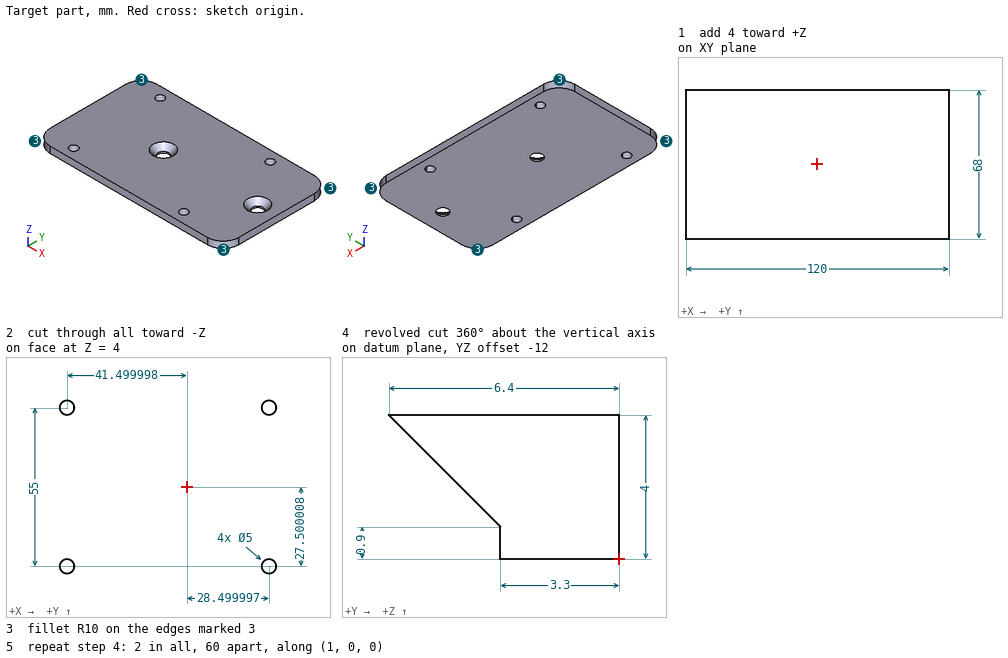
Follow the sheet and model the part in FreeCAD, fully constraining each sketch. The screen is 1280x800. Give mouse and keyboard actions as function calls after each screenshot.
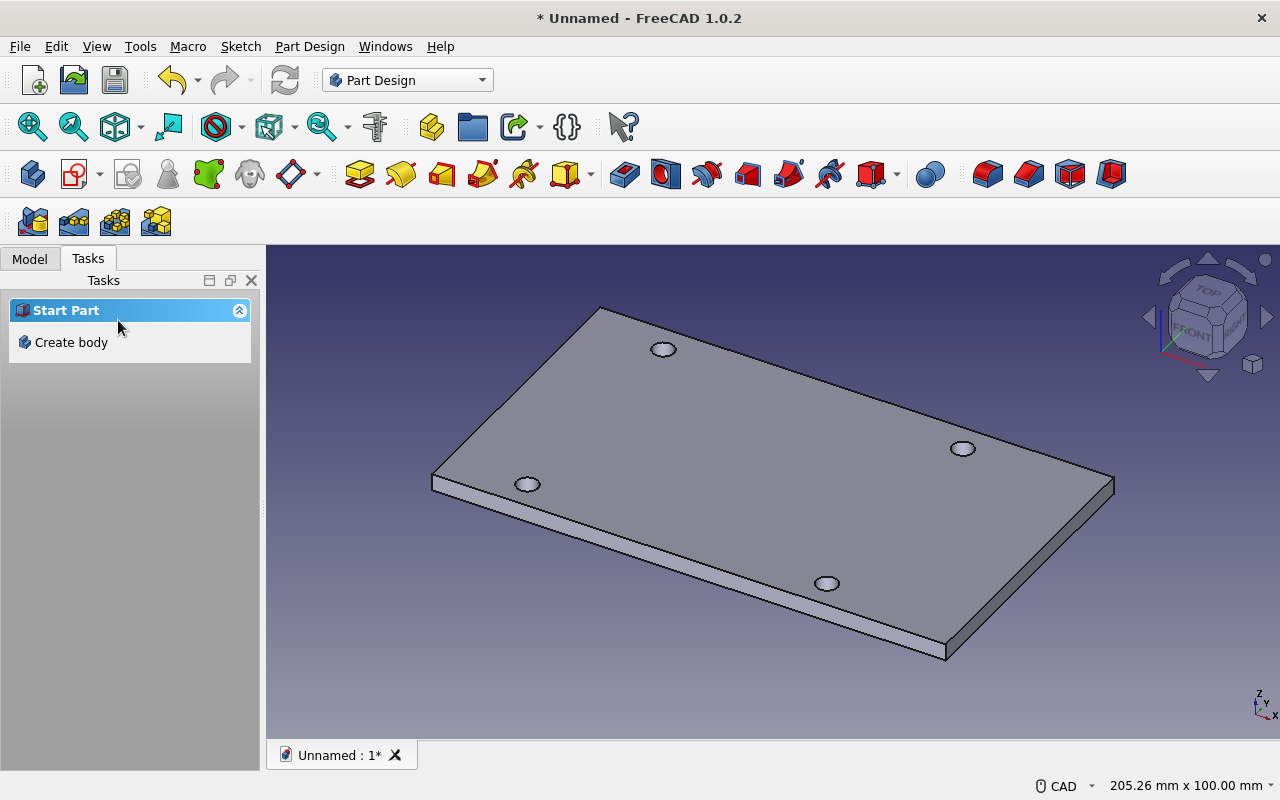
click(946, 651)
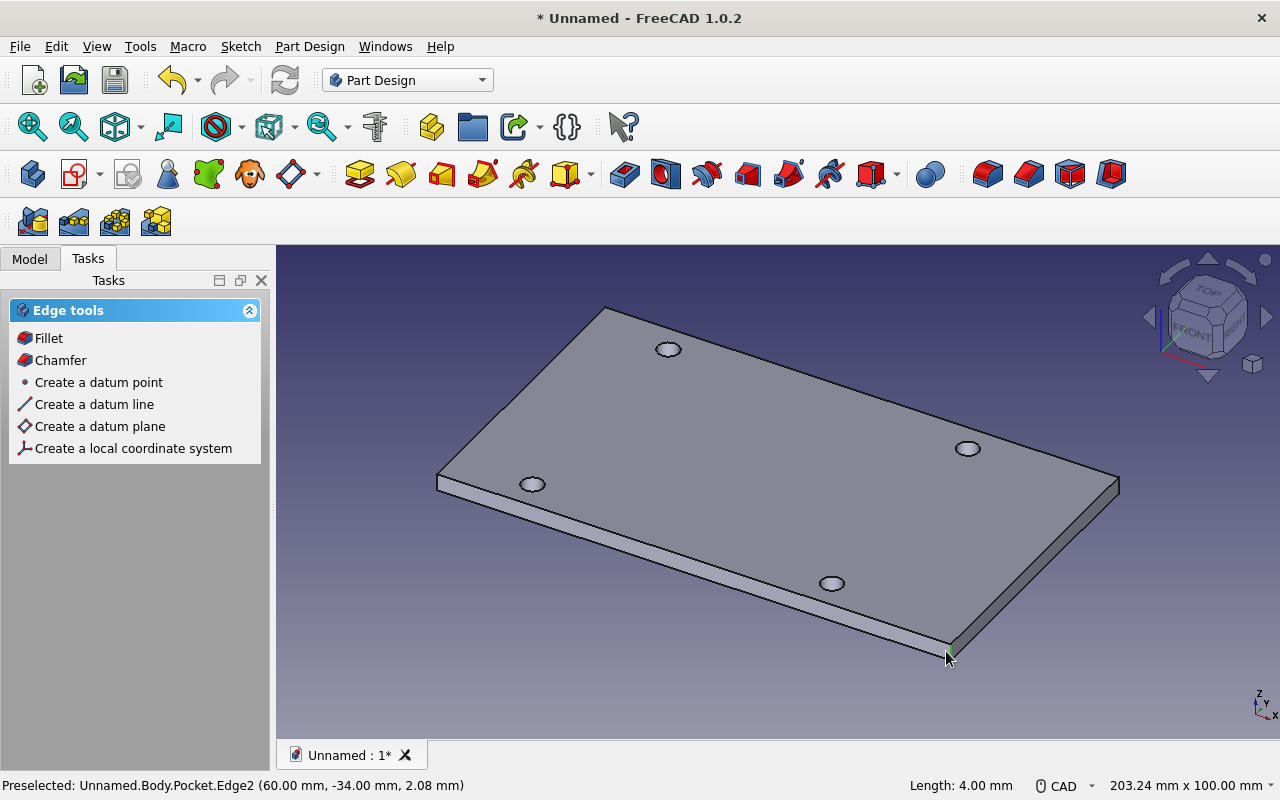
scroll(437, 481, up, 4)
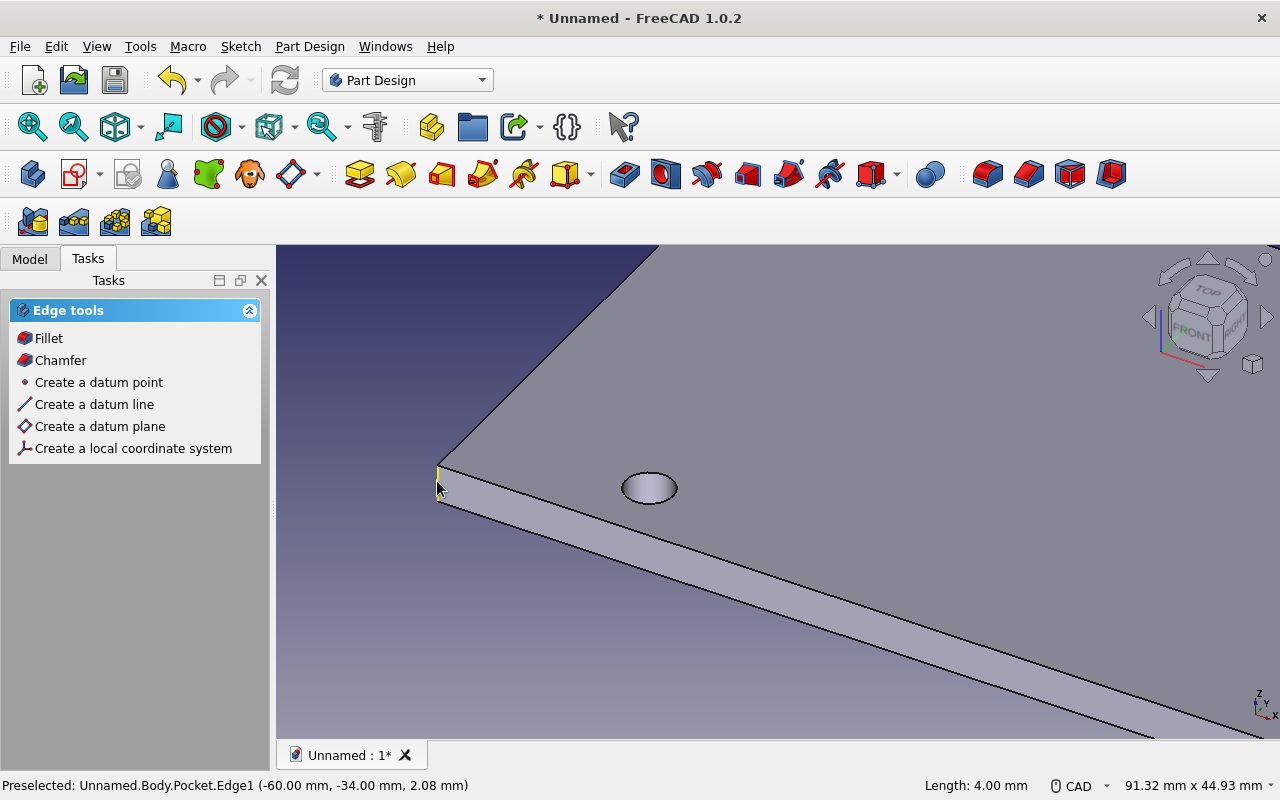
click(33, 128)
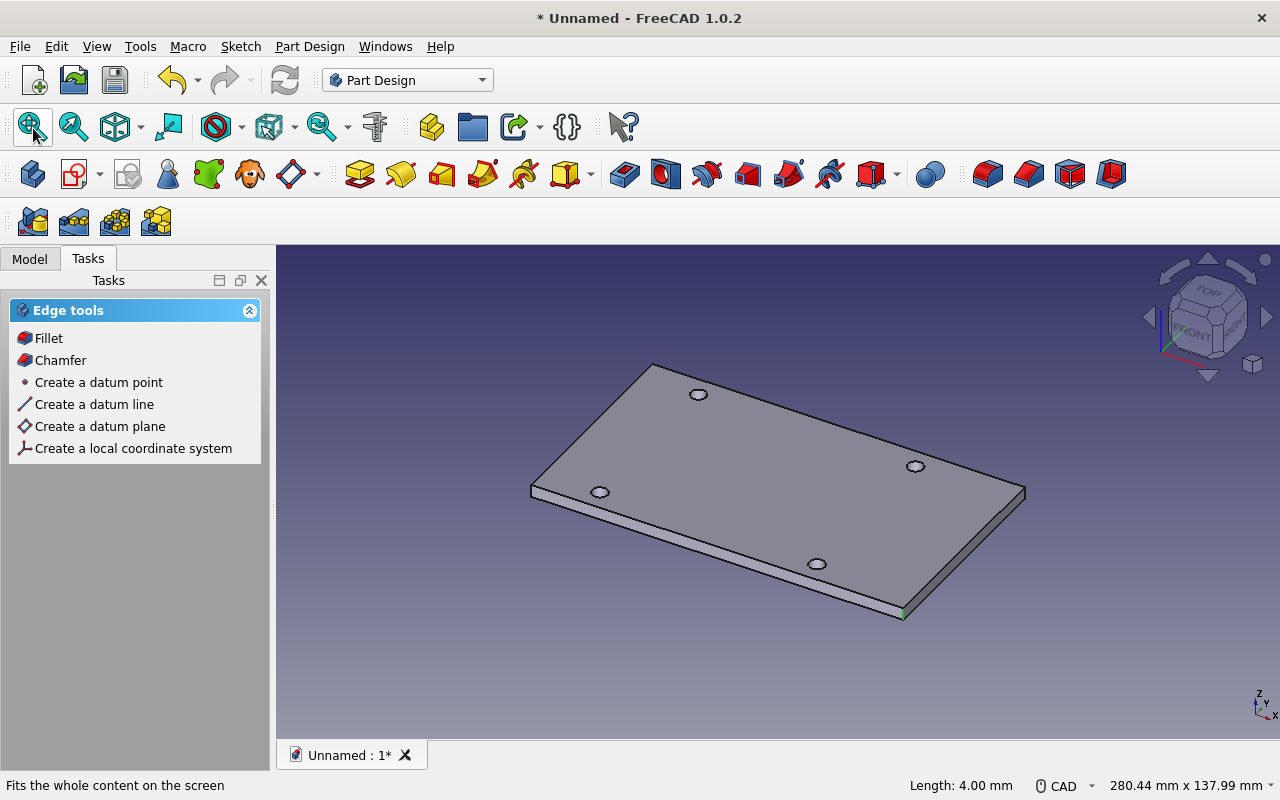
key(0)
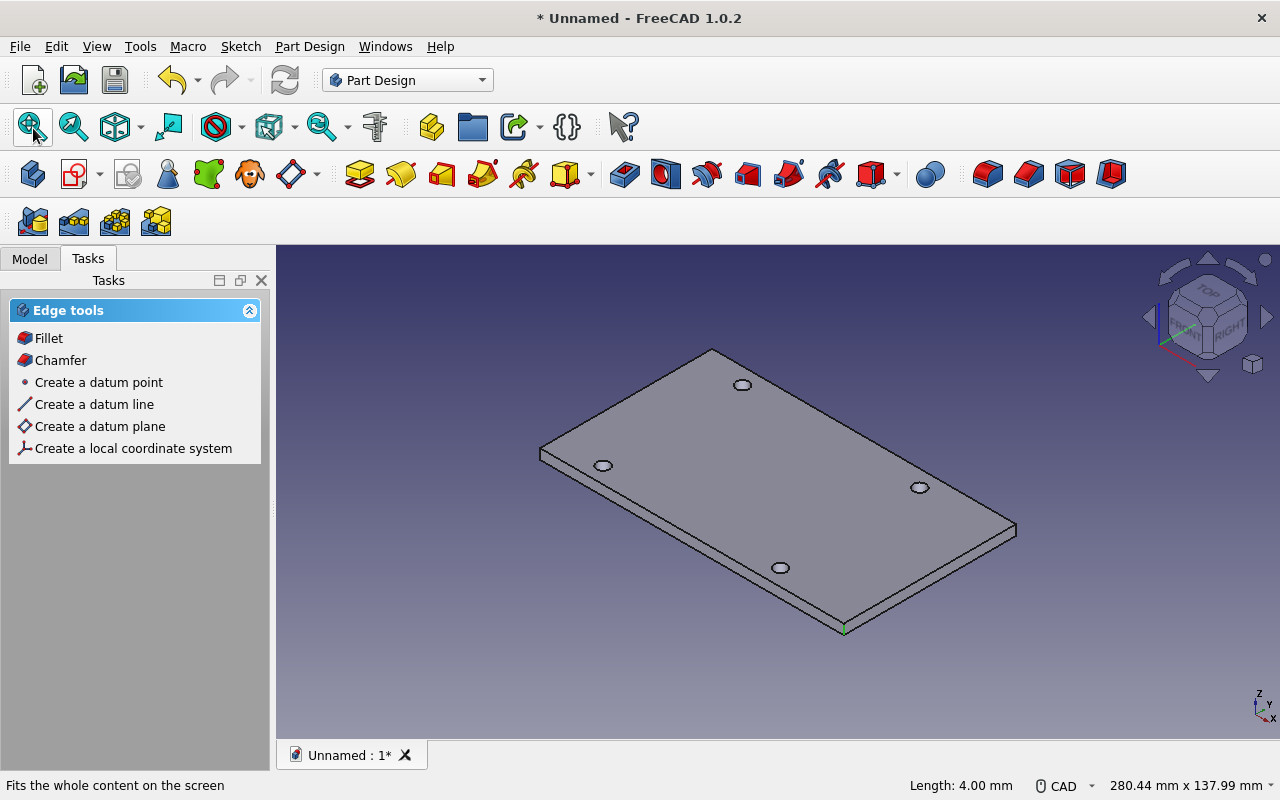
scroll(540, 453, up, 6)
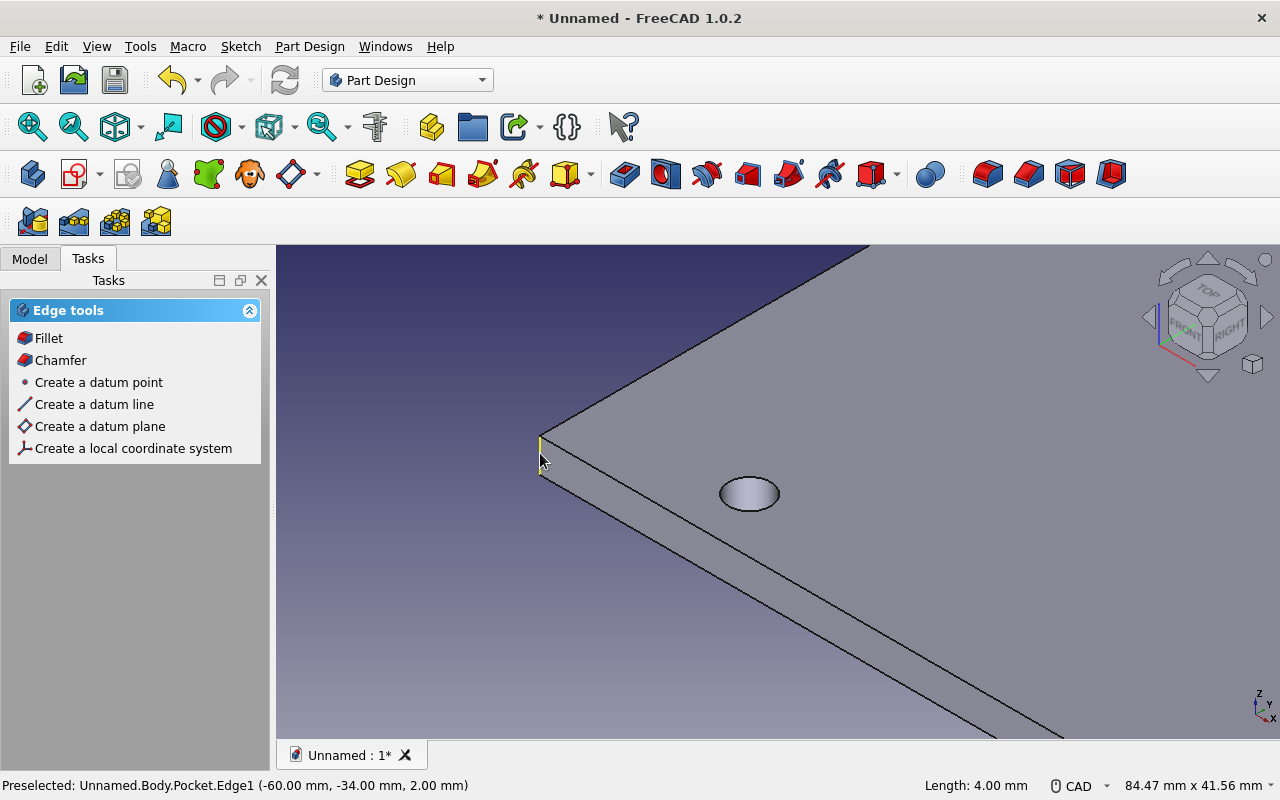
click(33, 128)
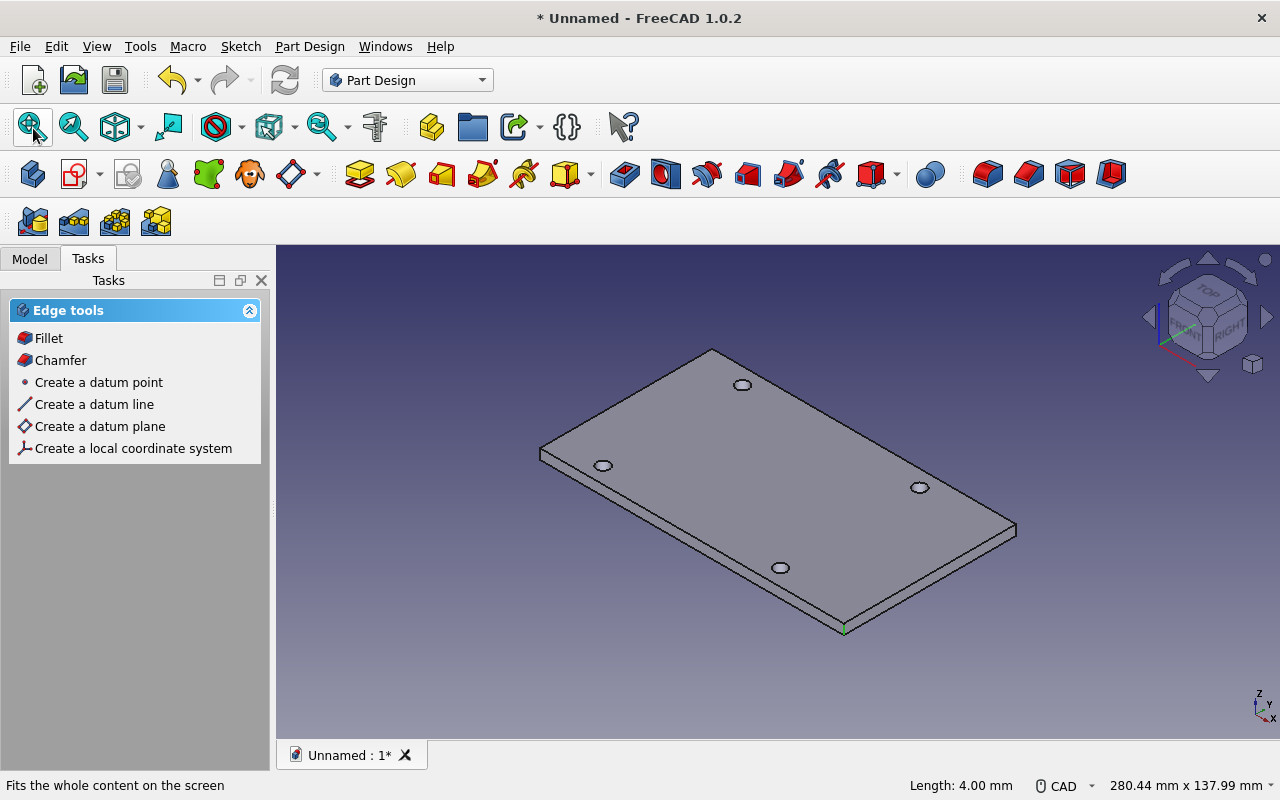
key(2)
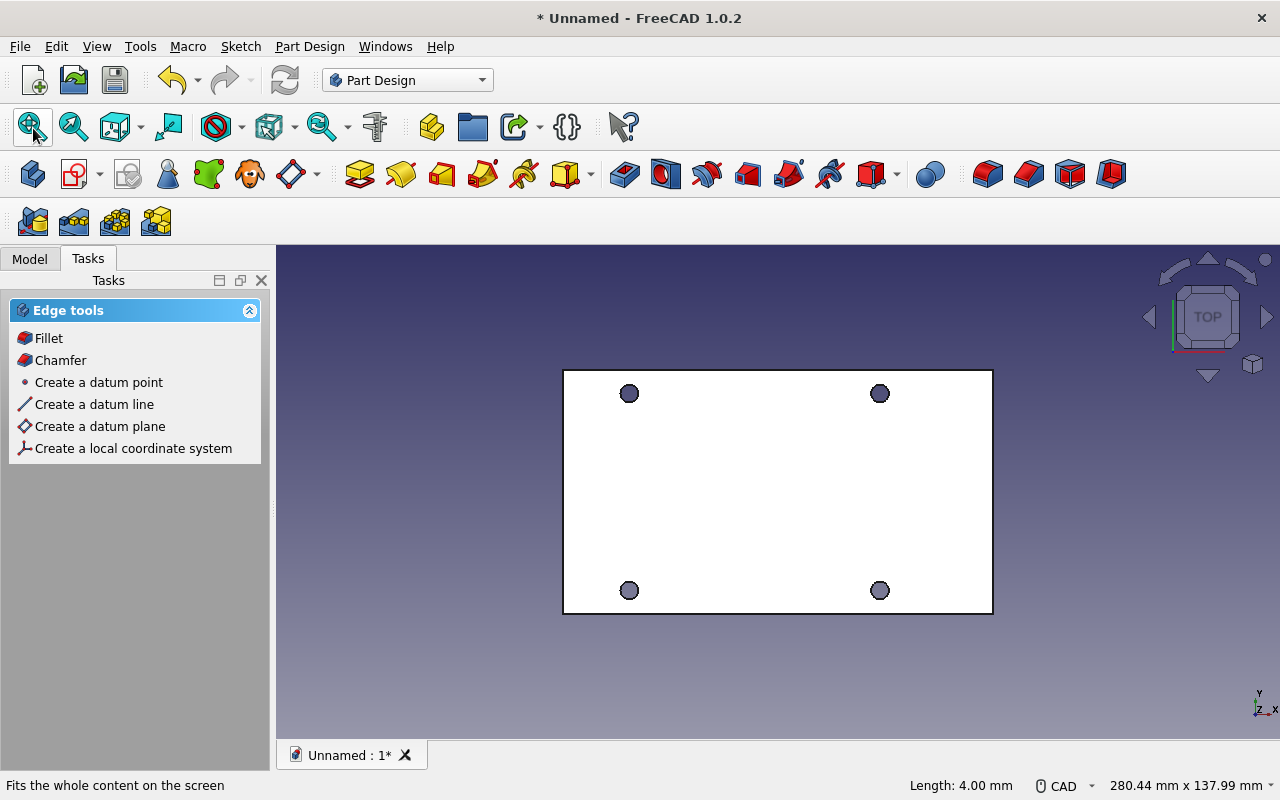
scroll(563, 613, up, 6)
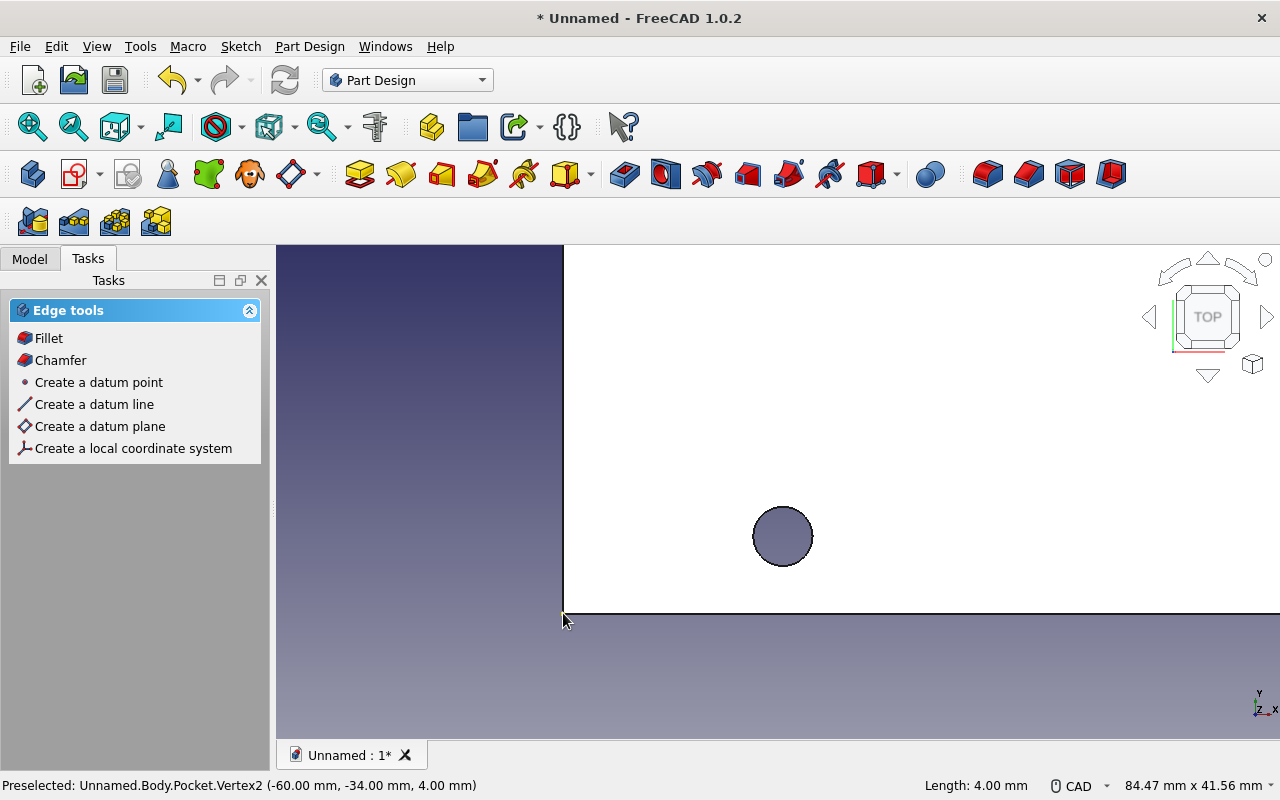
click(33, 128)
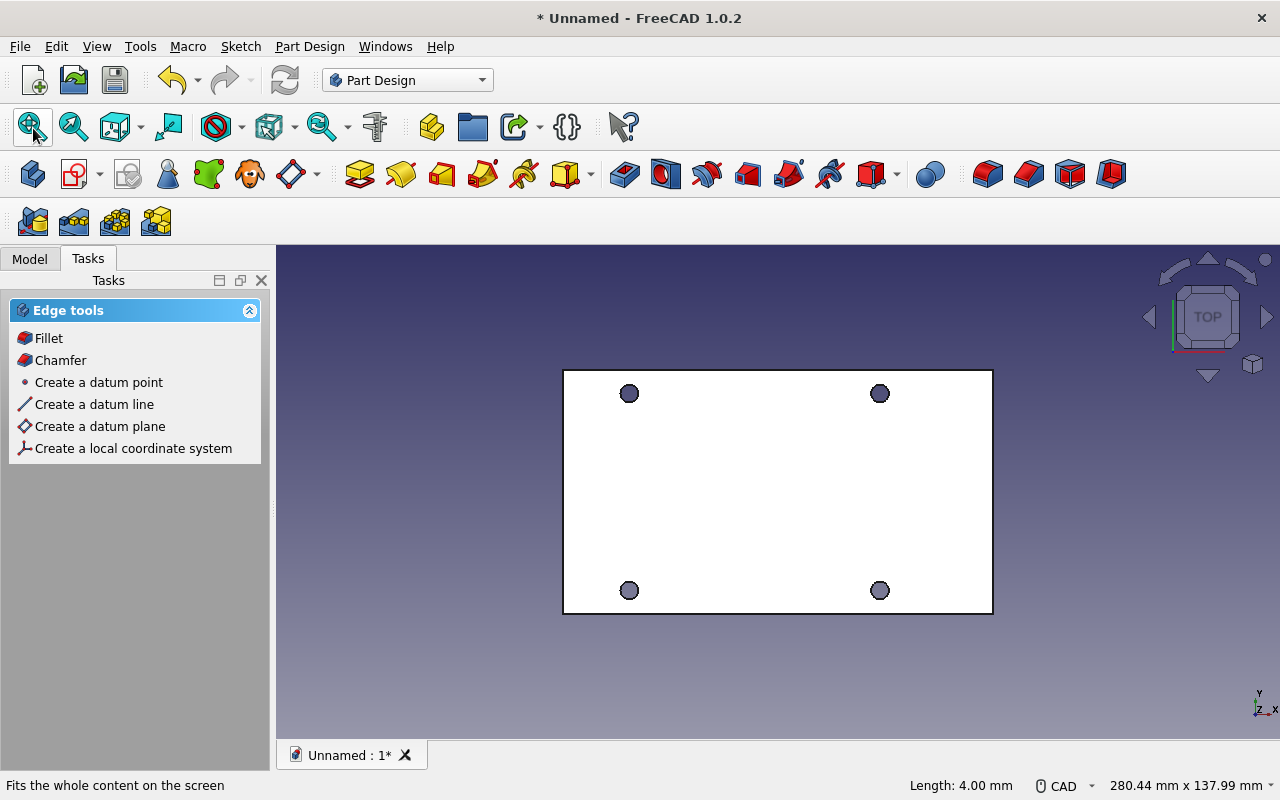
key(1)